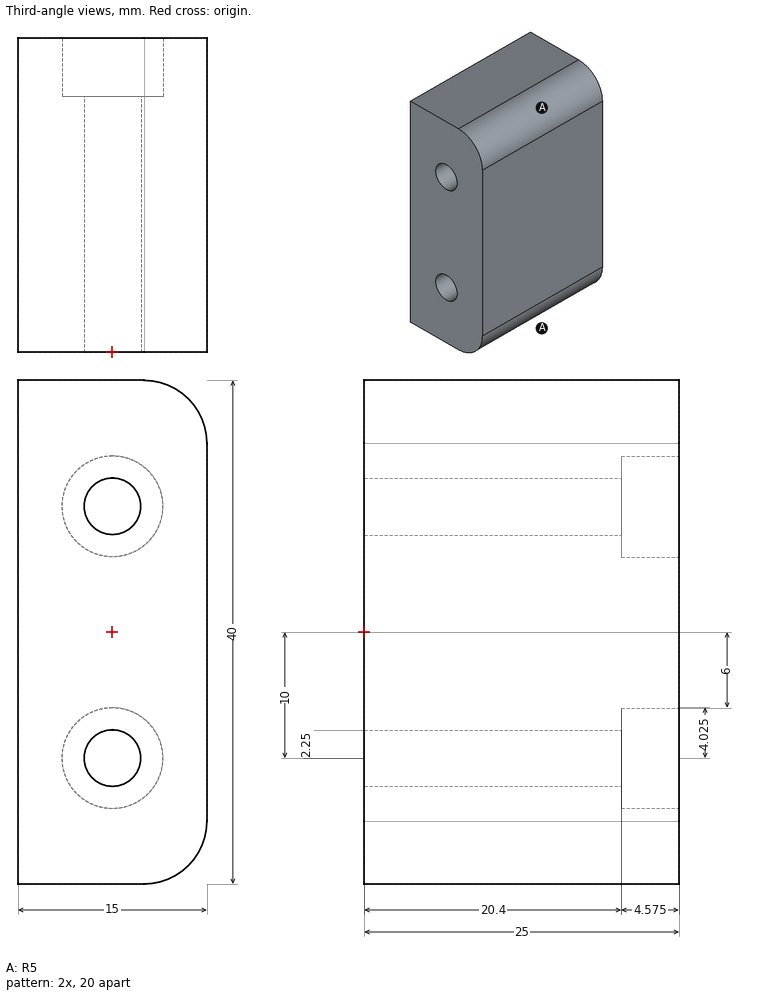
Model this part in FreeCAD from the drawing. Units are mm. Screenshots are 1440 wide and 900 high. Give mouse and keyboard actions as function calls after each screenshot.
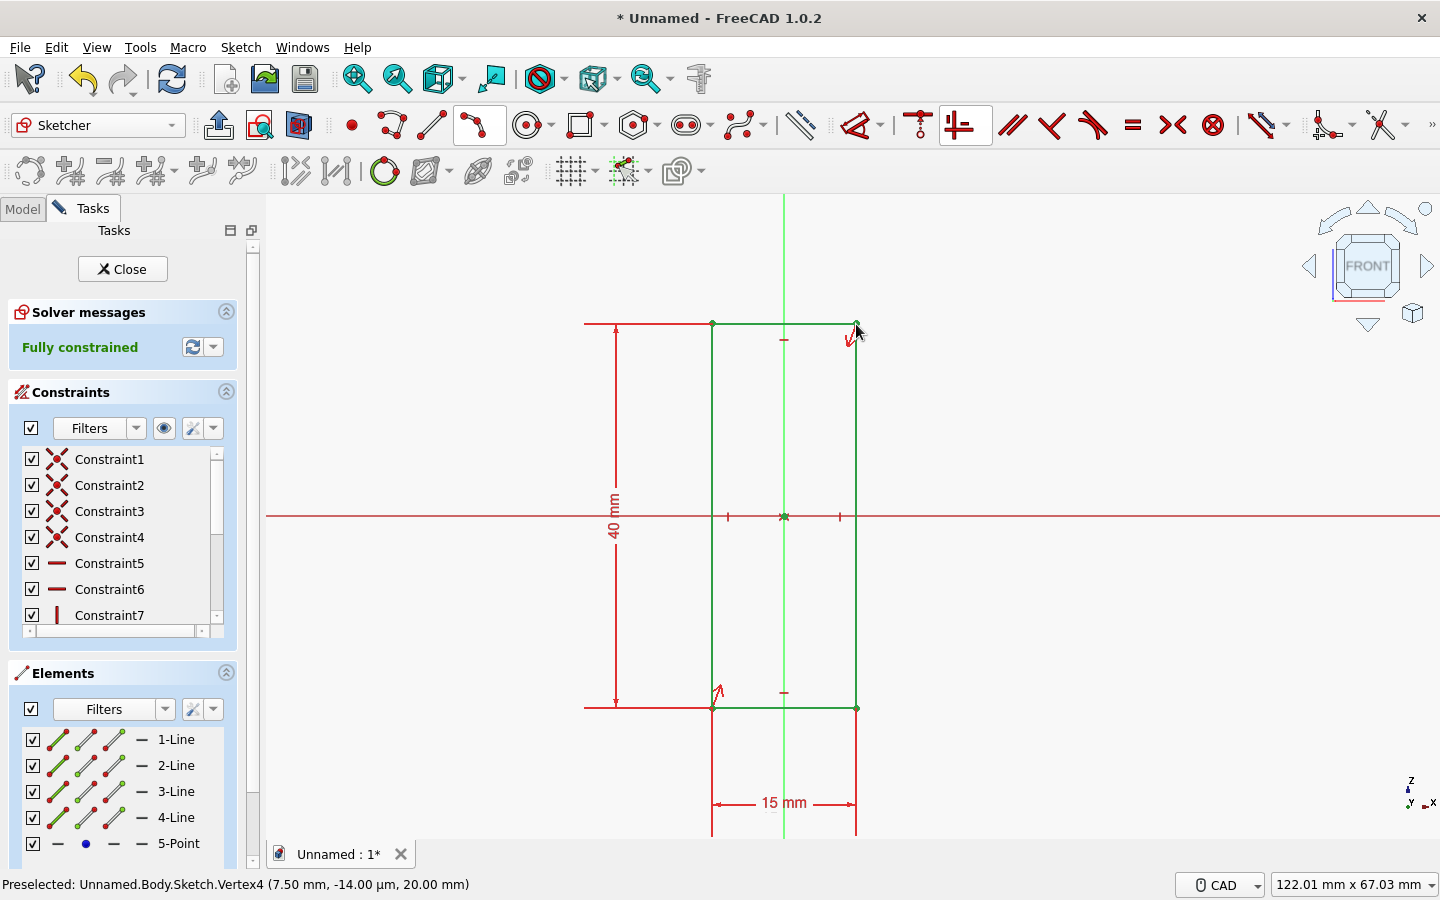
click(123, 269)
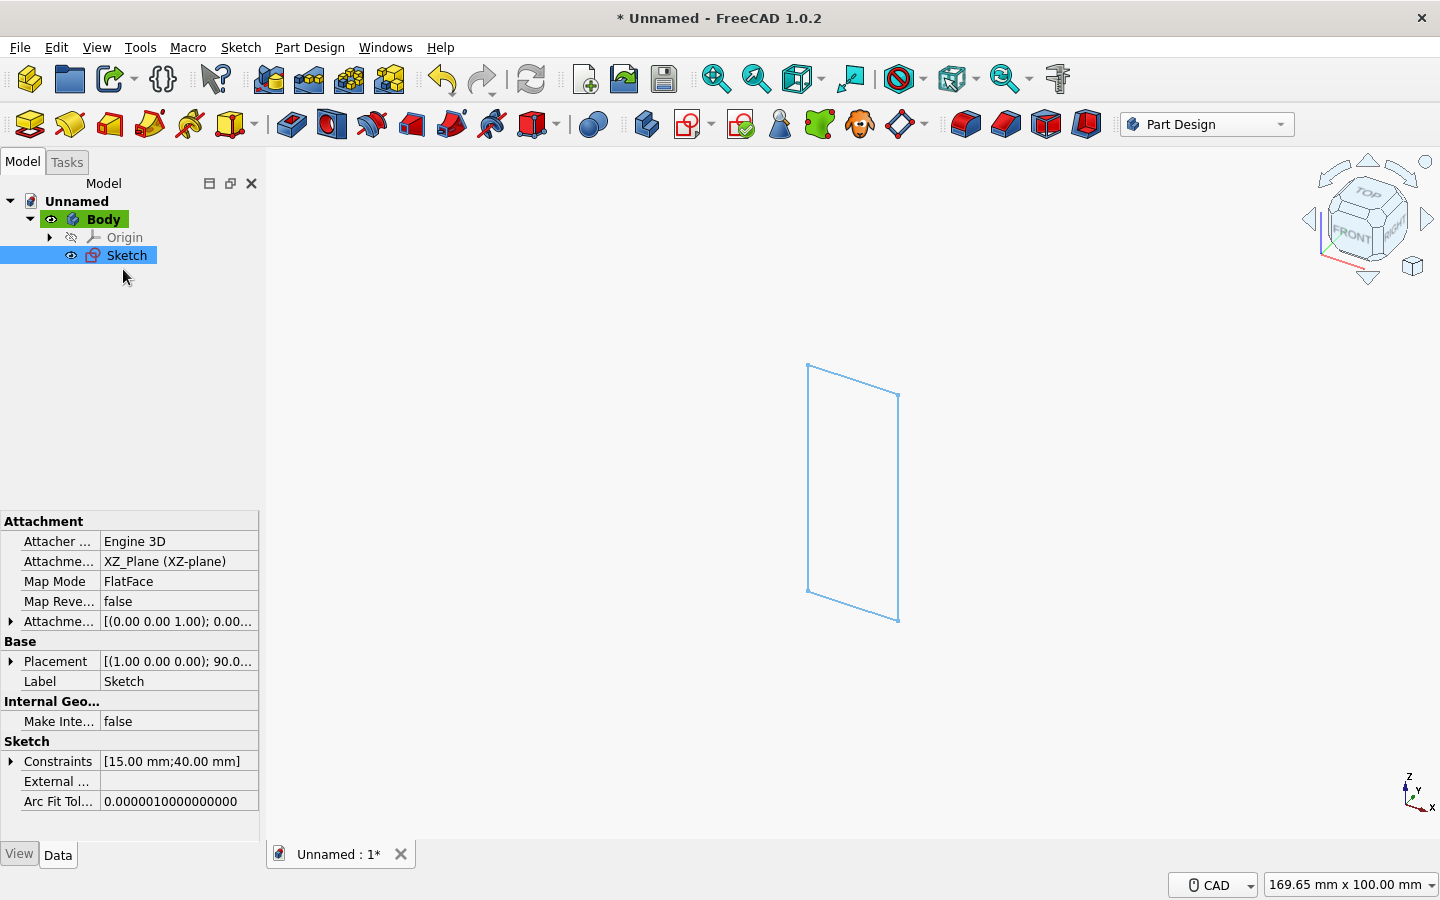
click(30, 124)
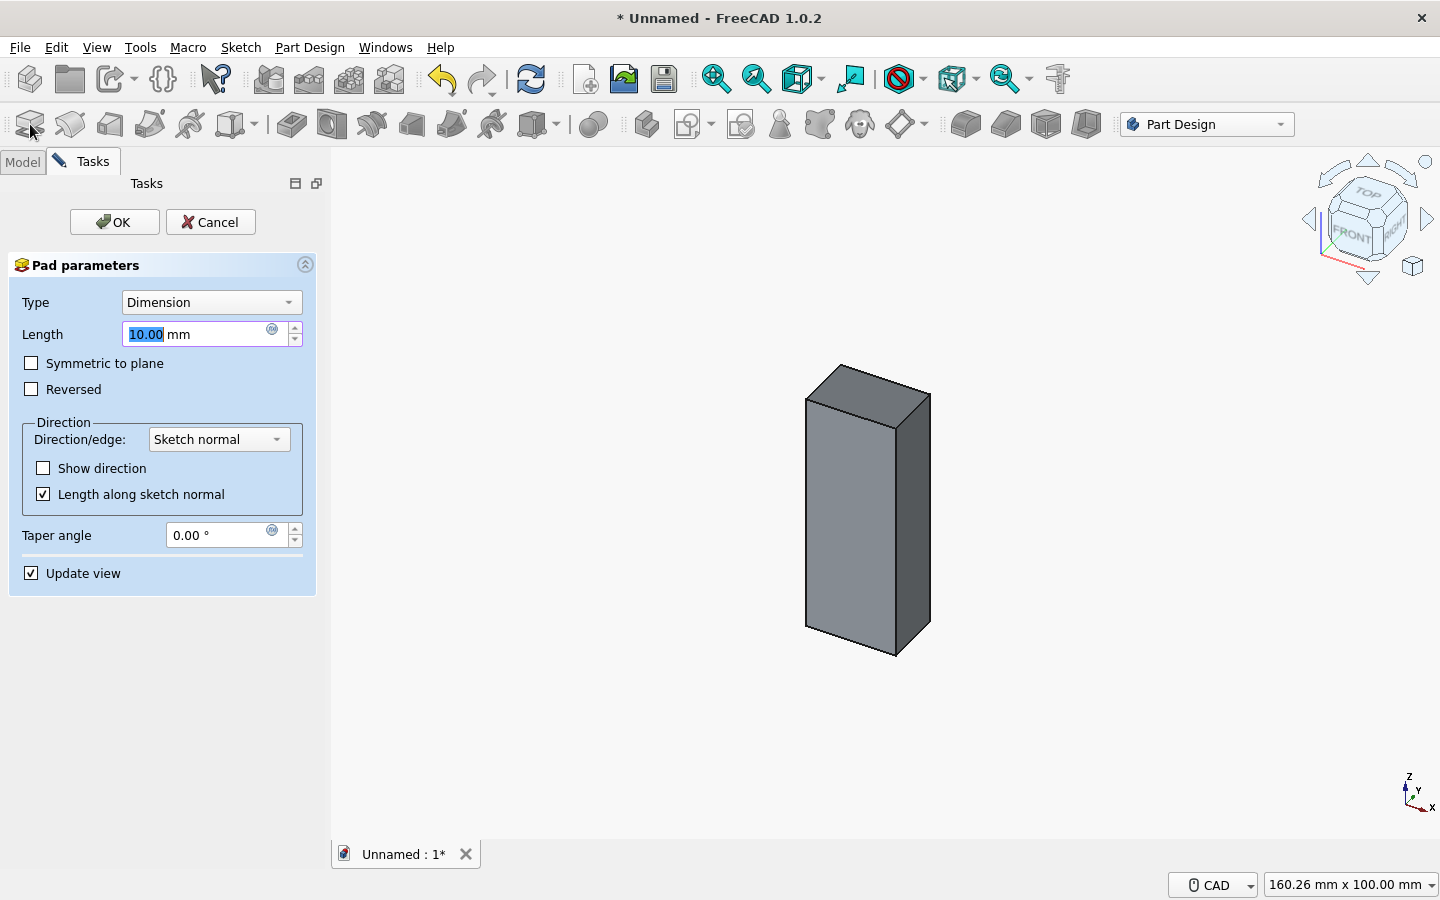
text(25)
key(Tab)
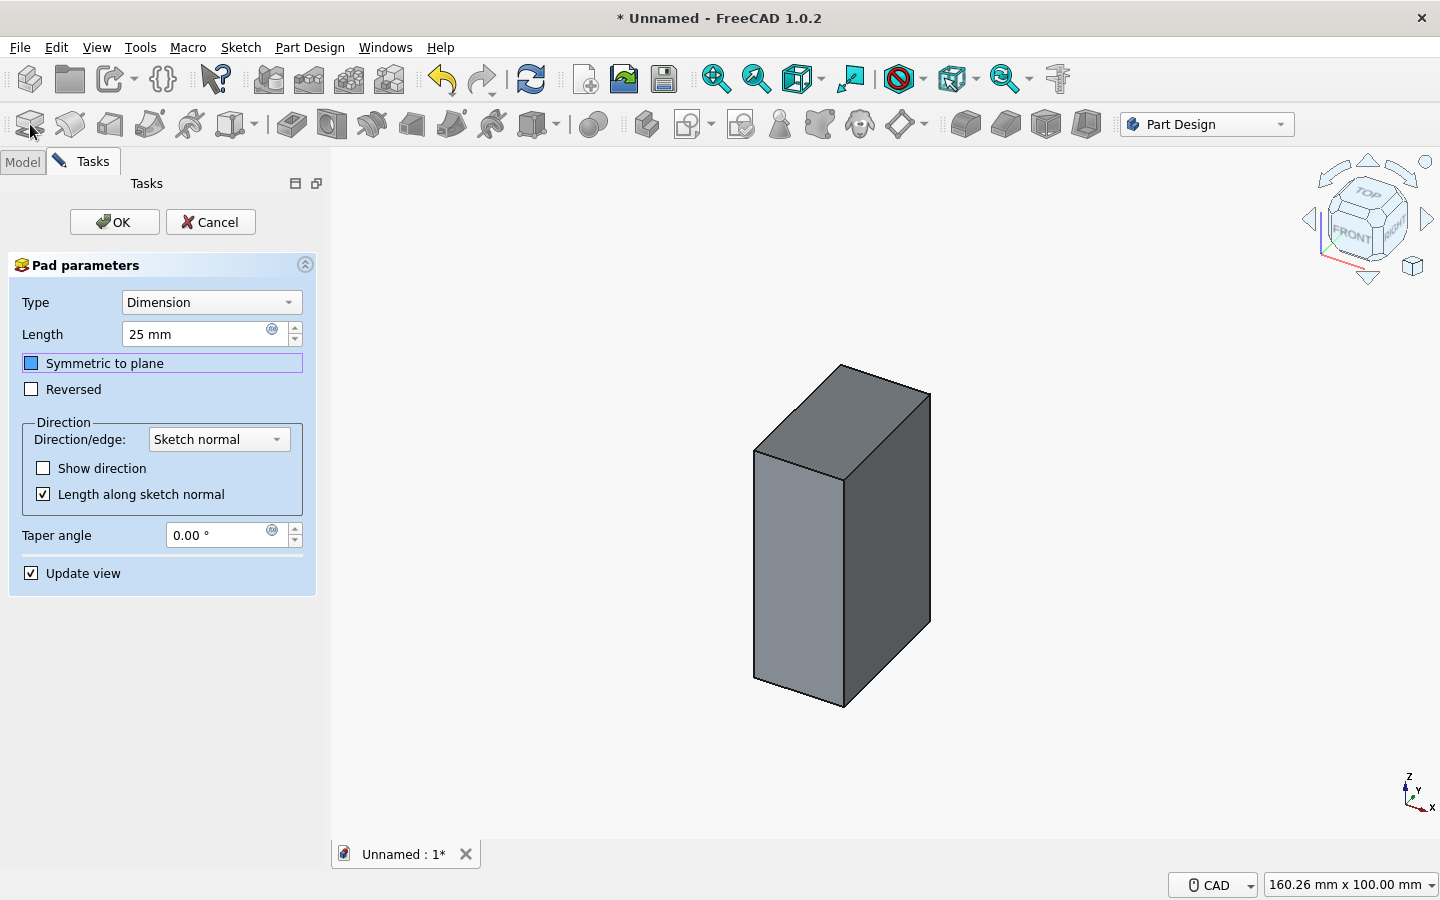
click(30, 389)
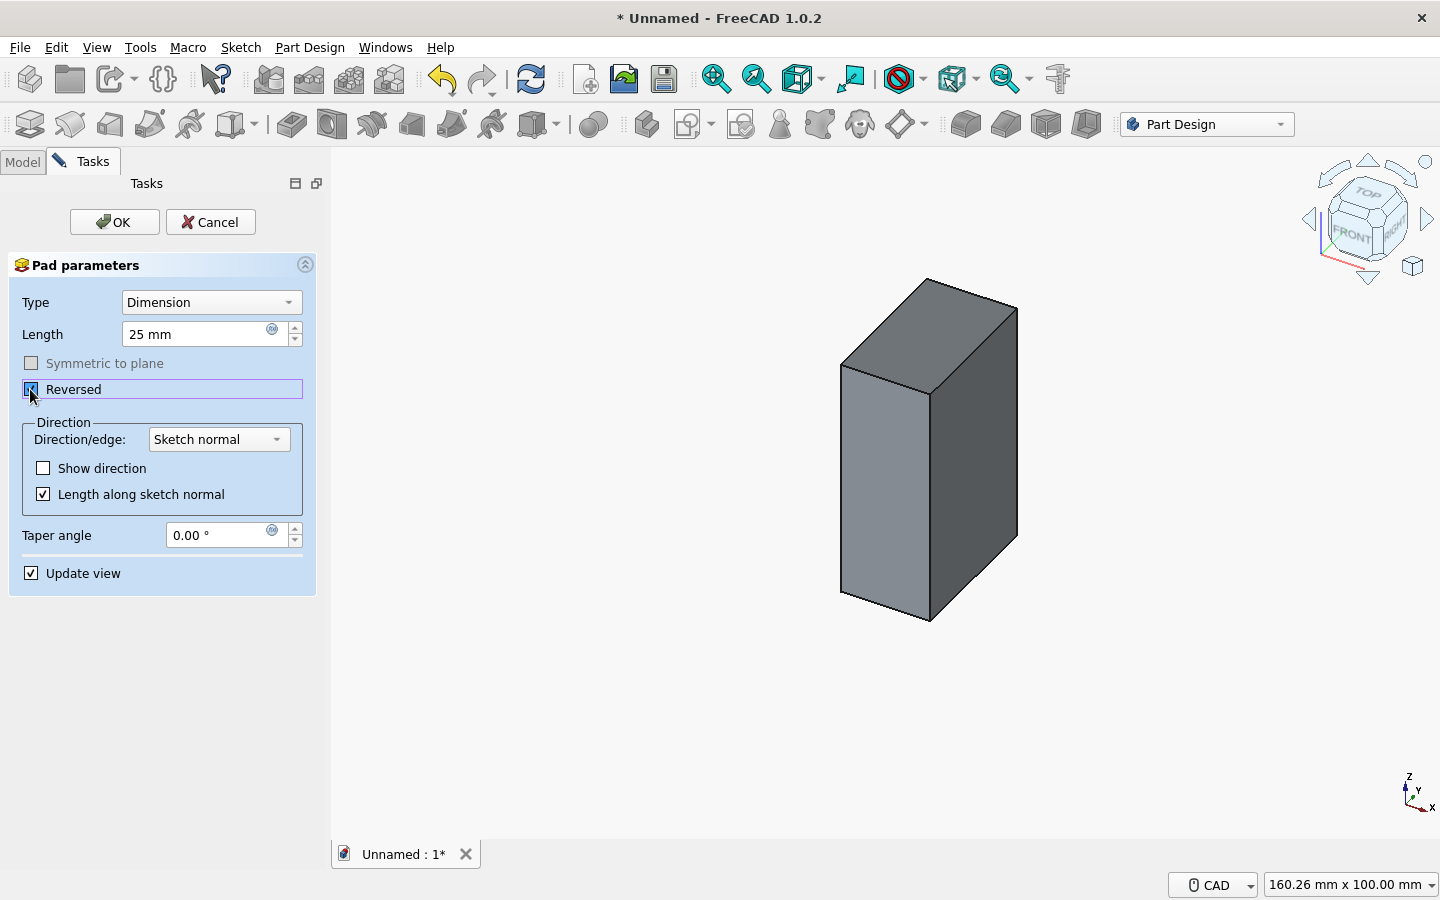
click(115, 222)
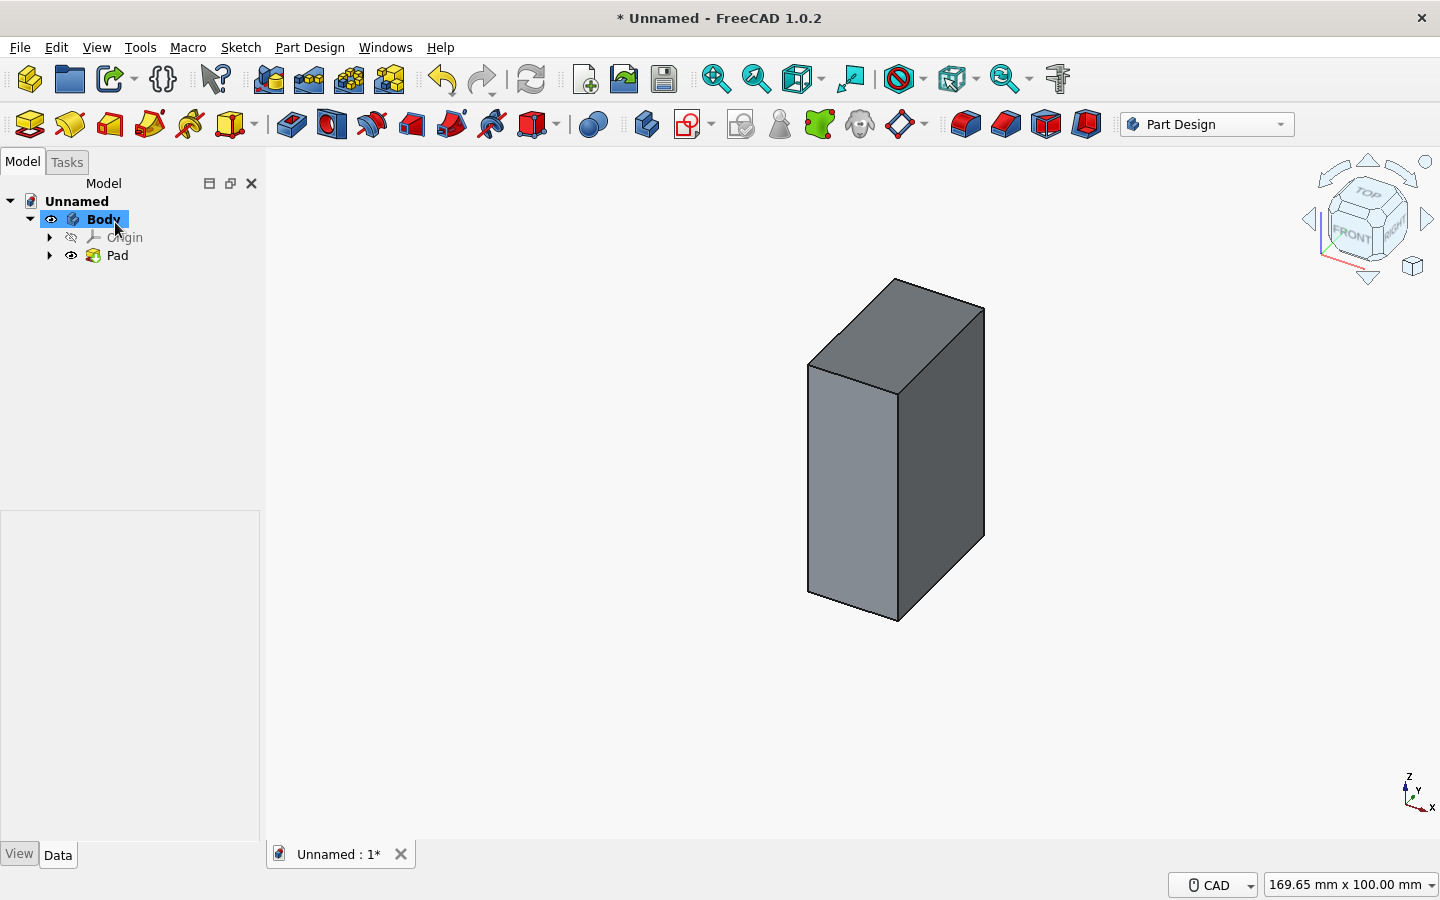
click(941, 351)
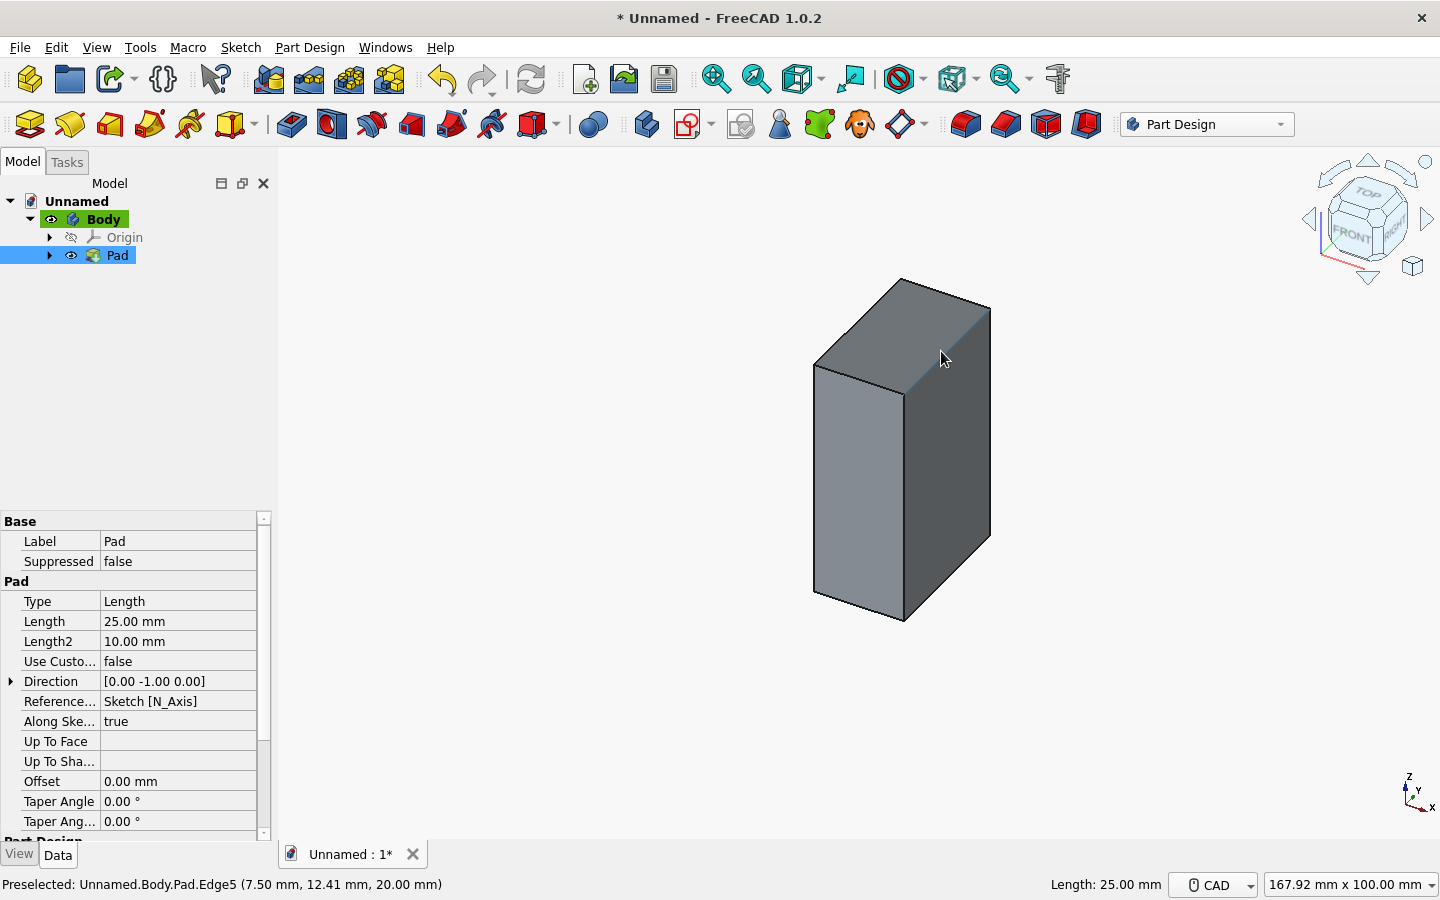
key(0)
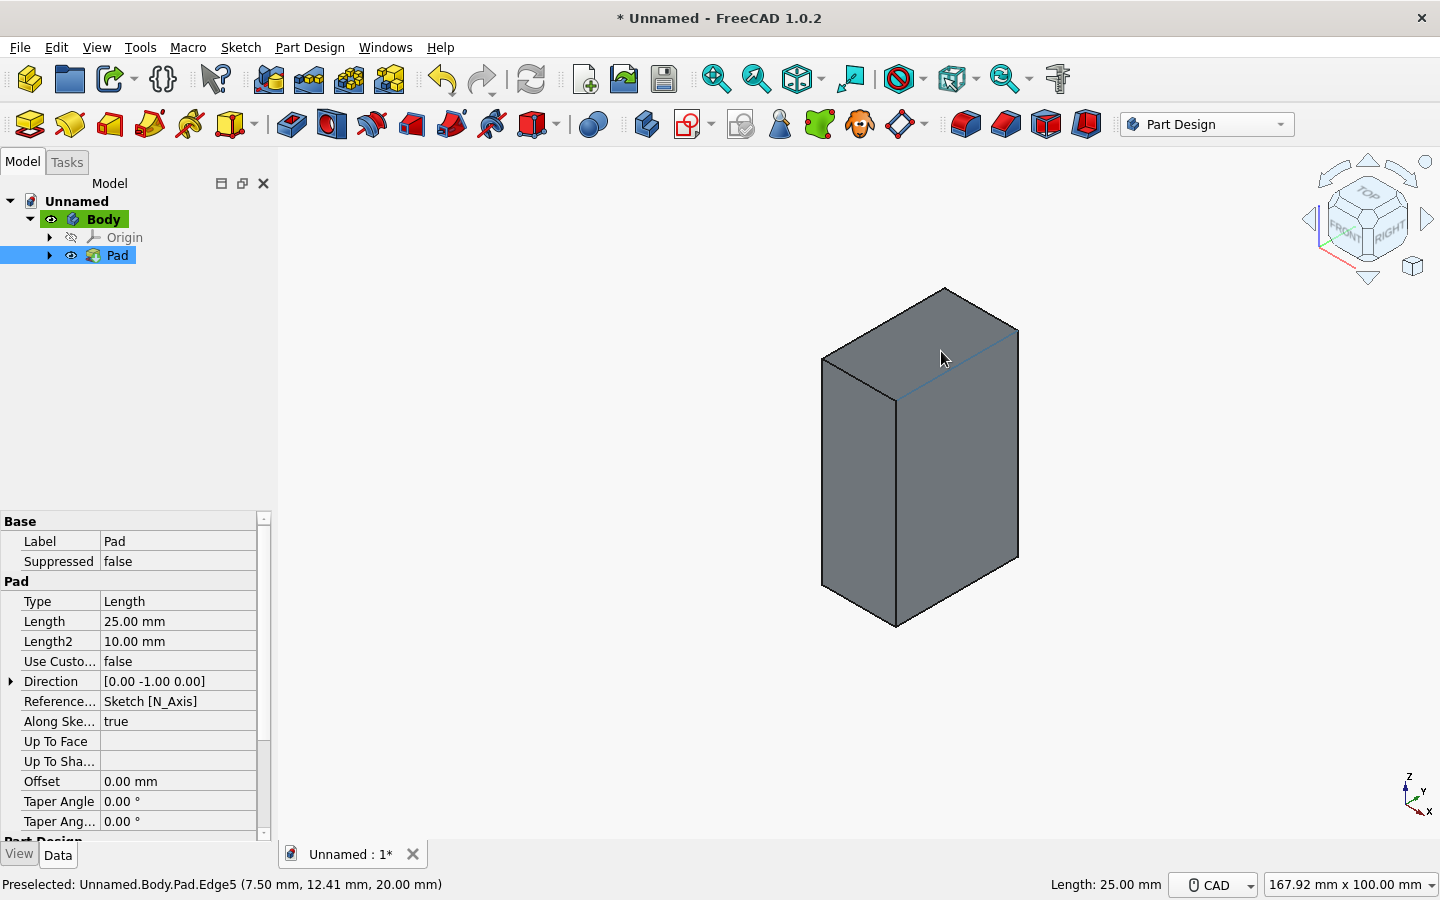
key(2)